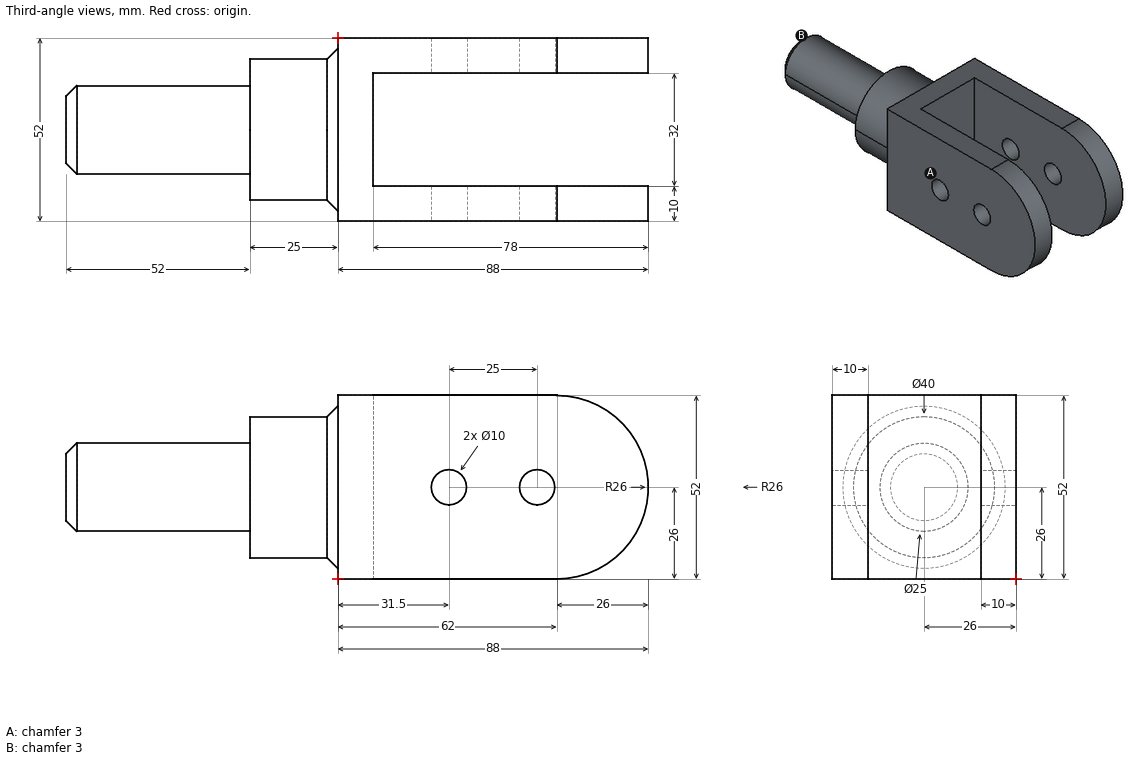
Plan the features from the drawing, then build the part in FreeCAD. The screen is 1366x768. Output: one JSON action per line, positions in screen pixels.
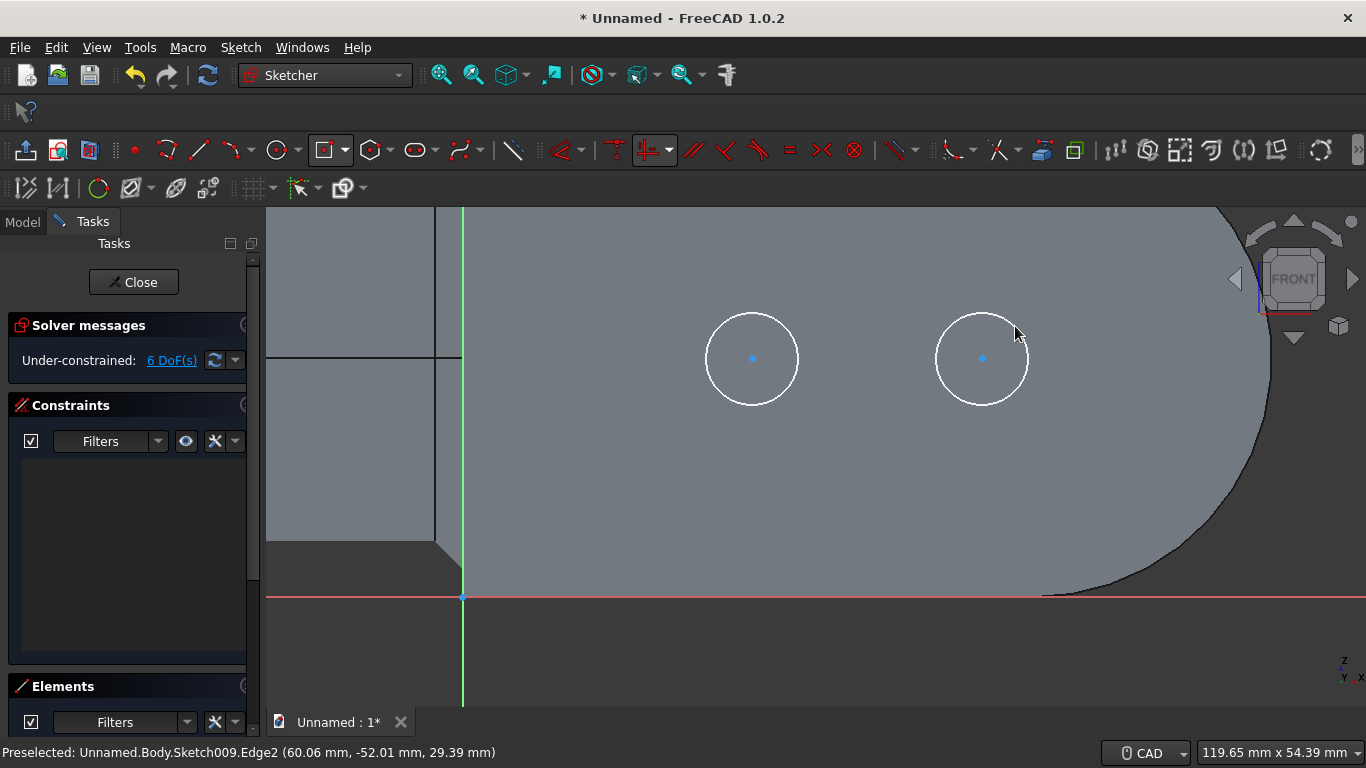
{"action": "left_click", "coordinate": [784, 326]}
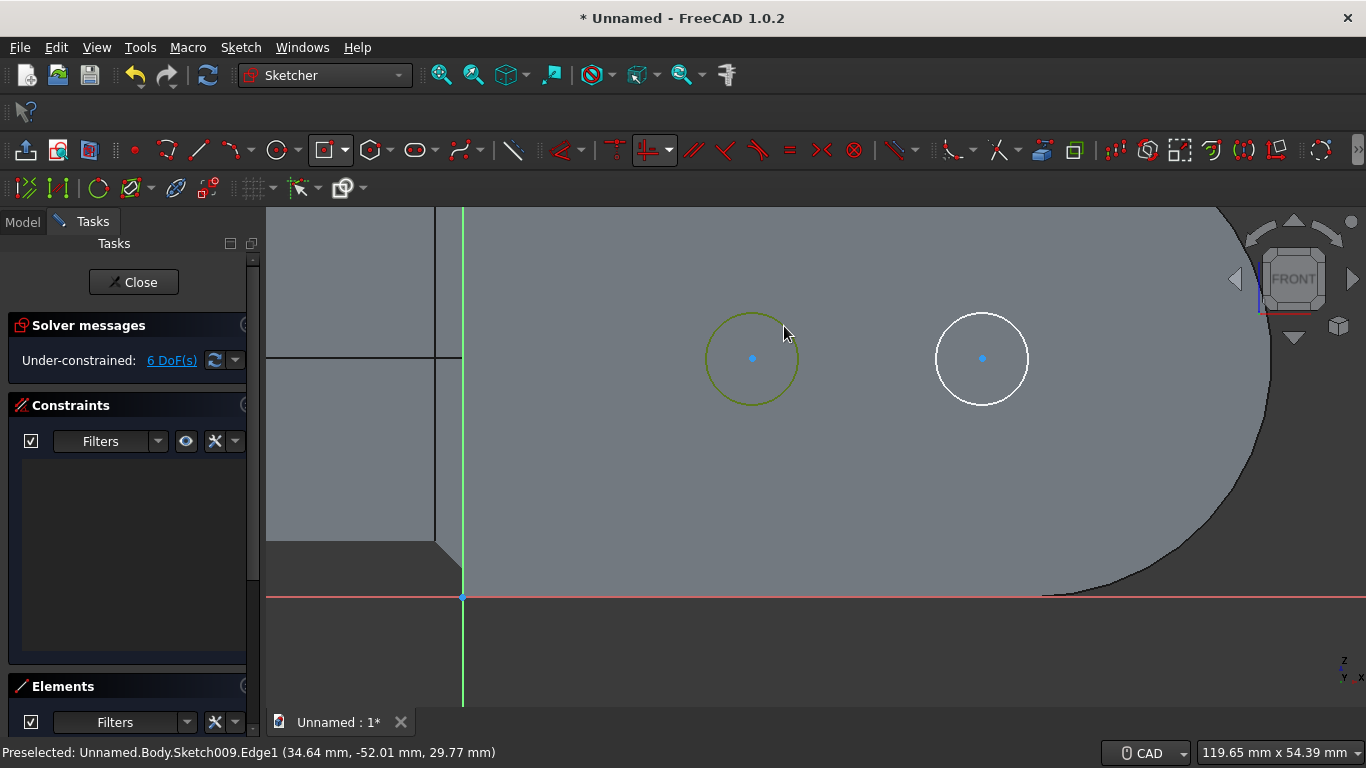
{"action": "left_click", "coordinate": [1014, 326]}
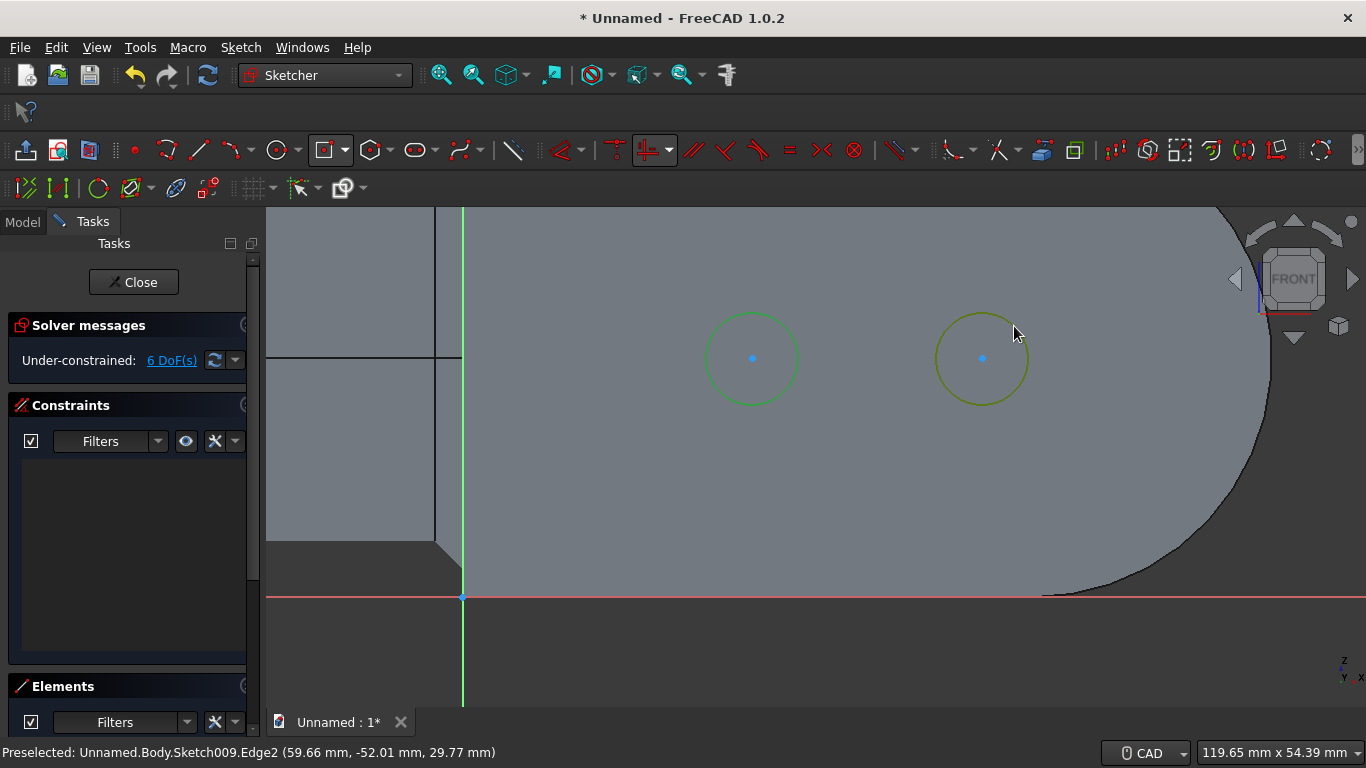
{"action": "left_click", "coordinate": [790, 150]}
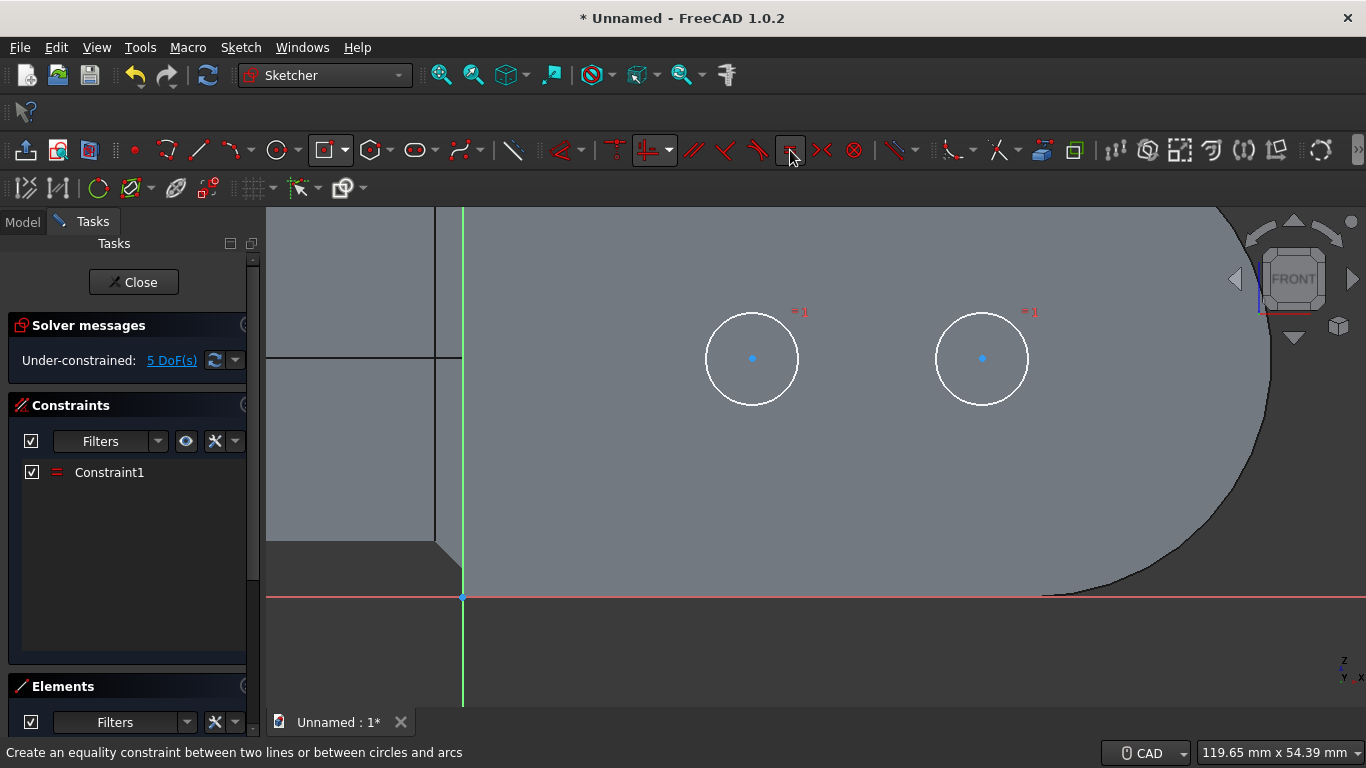
{"action": "left_click", "coordinate": [752, 359]}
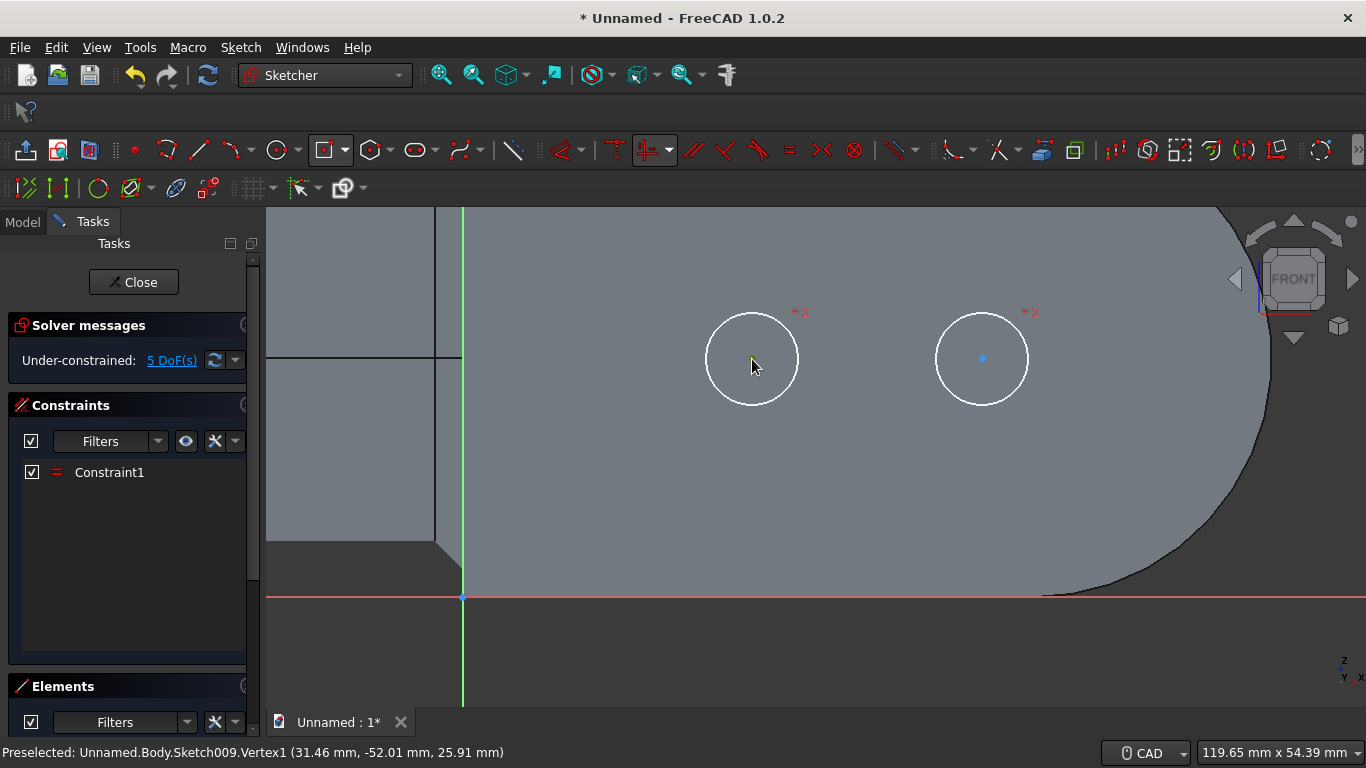
{"action": "left_click", "coordinate": [982, 359]}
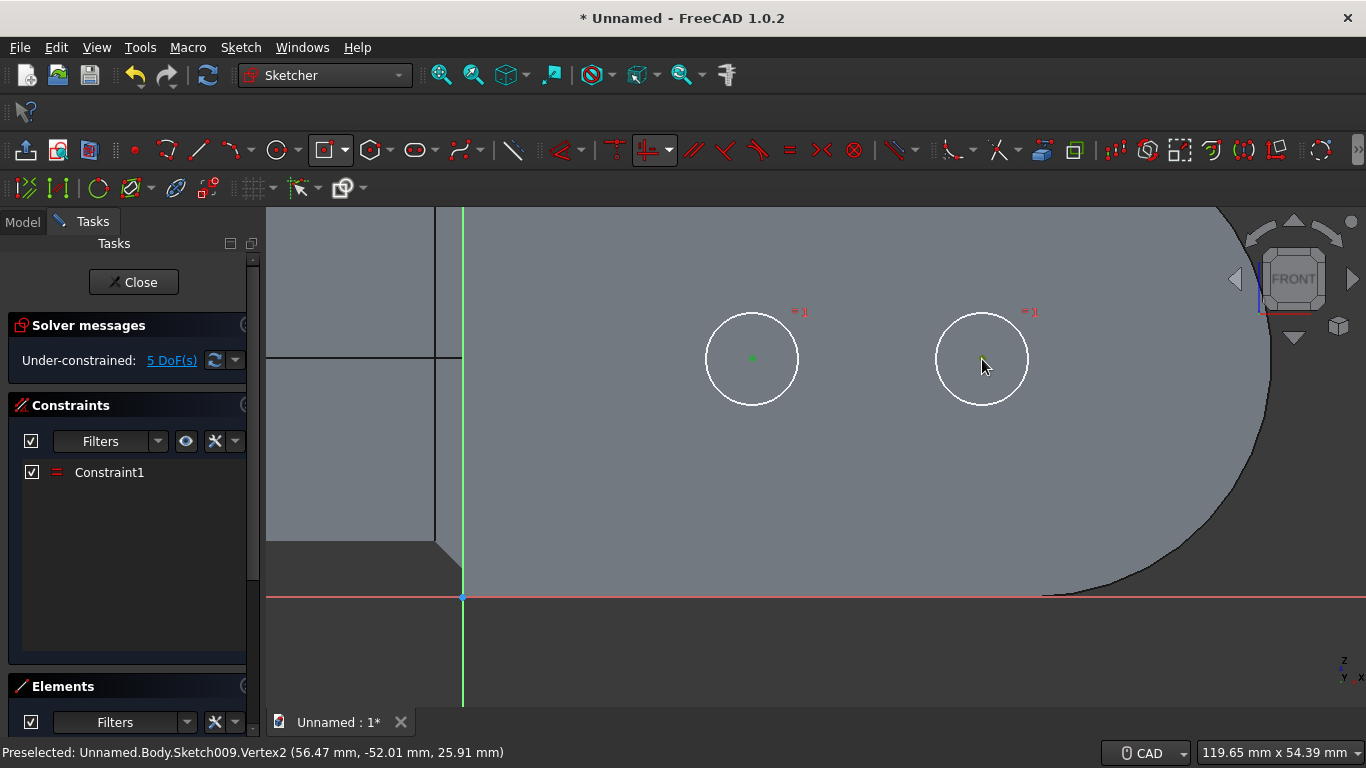
{"action": "left_click", "coordinate": [672, 150]}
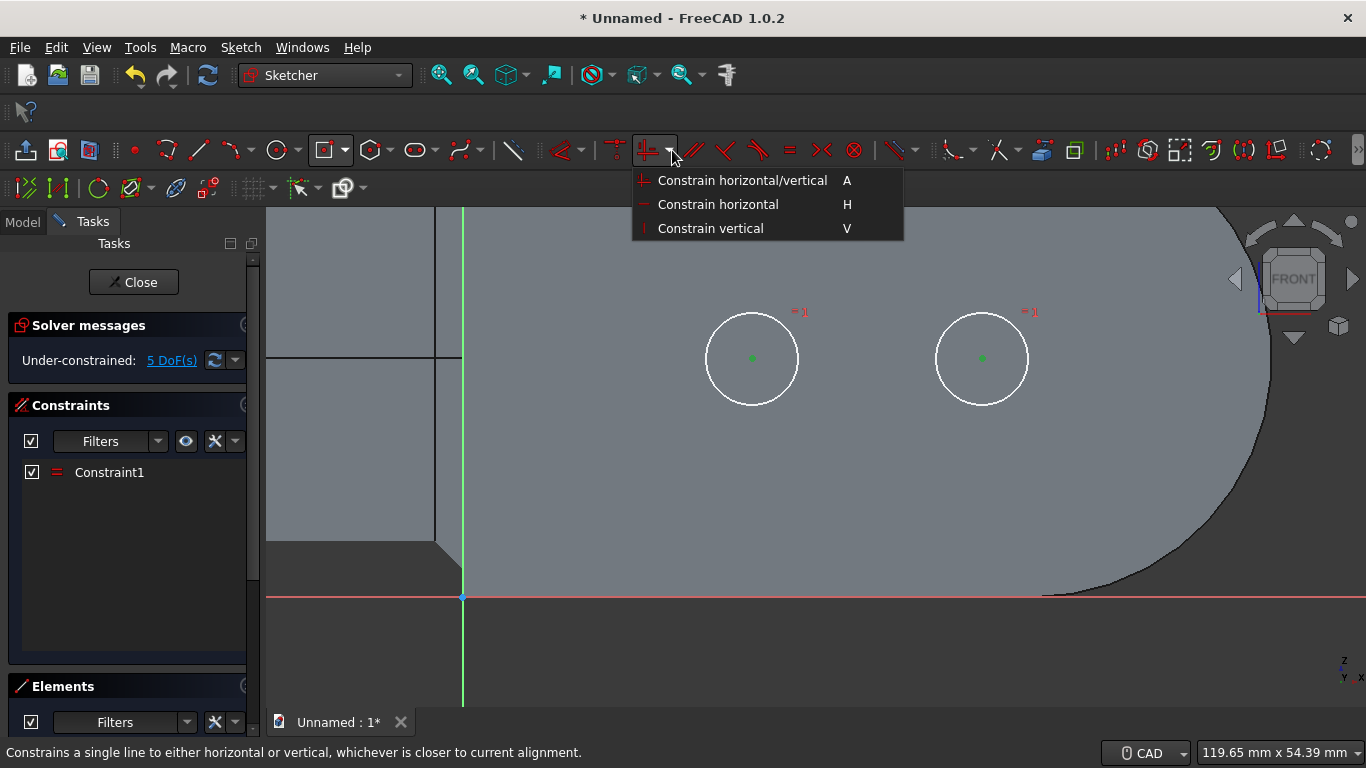
{"action": "left_click", "coordinate": [768, 204]}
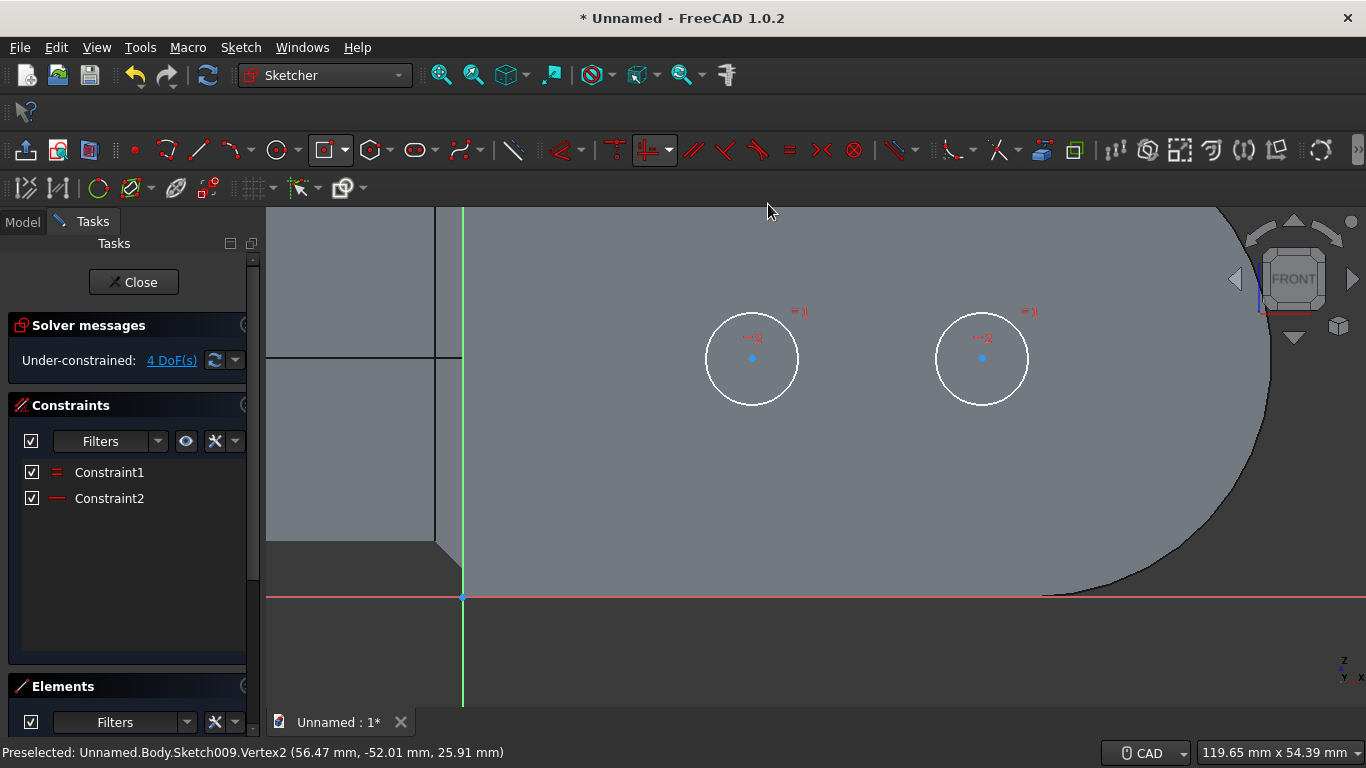
{"action": "left_click", "coordinate": [560, 150]}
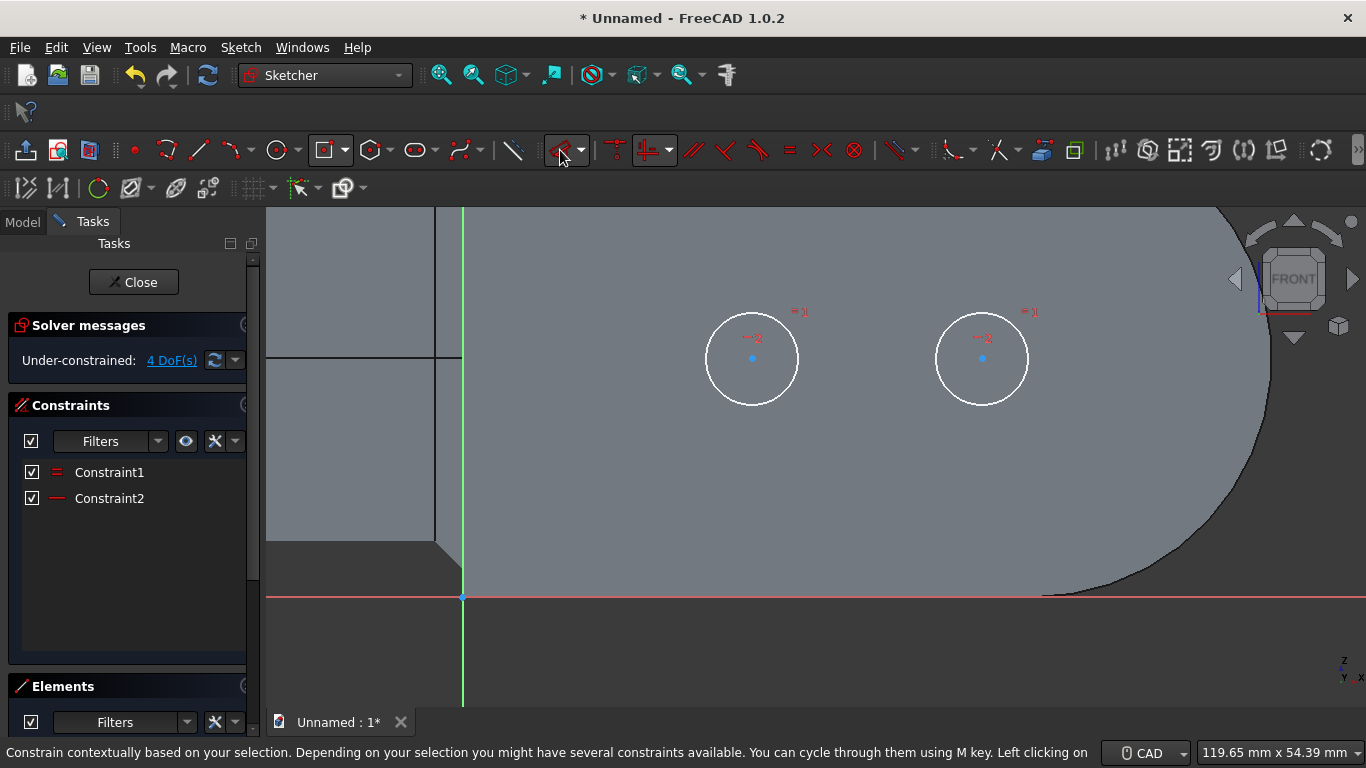
{"action": "left_click", "coordinate": [784, 326]}
{"action": "left_click", "coordinate": [806, 303]}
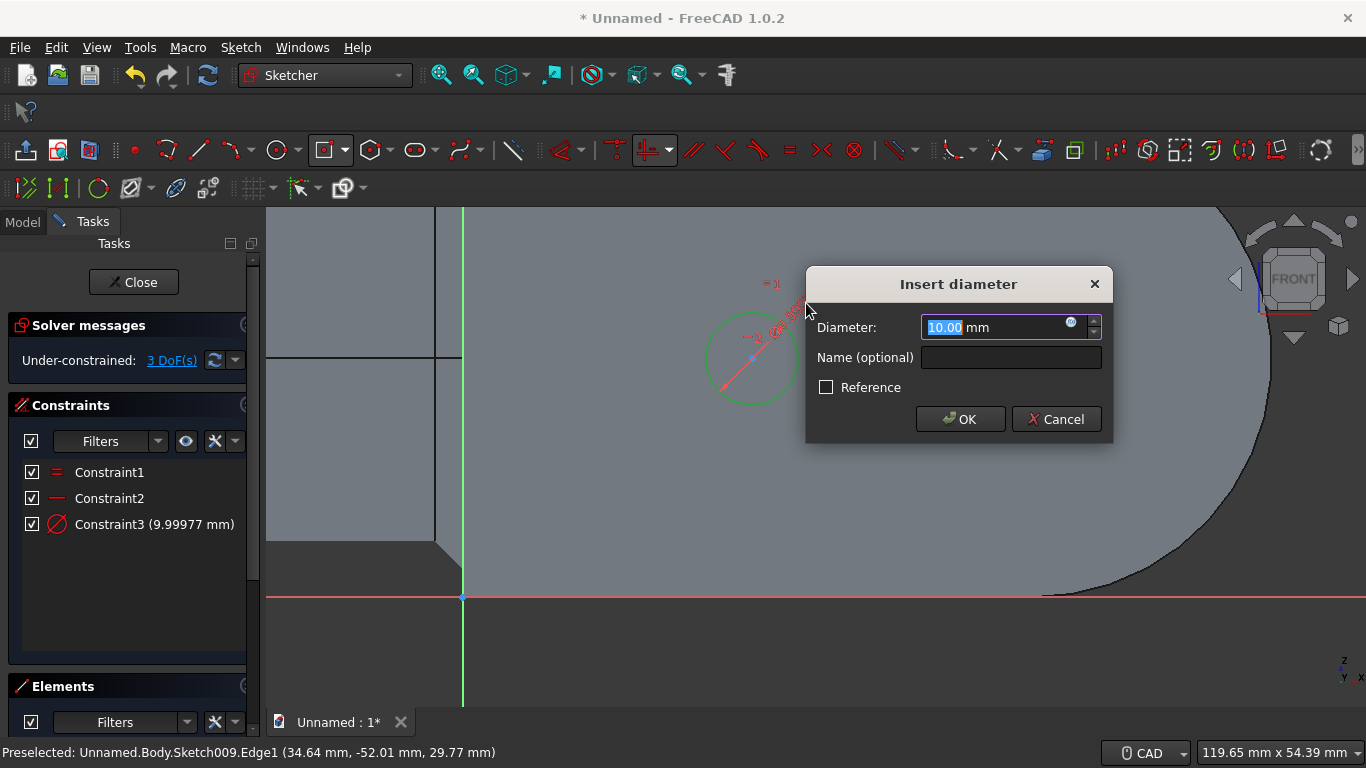
{"action": "type", "text": "10"}
{"action": "key", "text": "Return"}